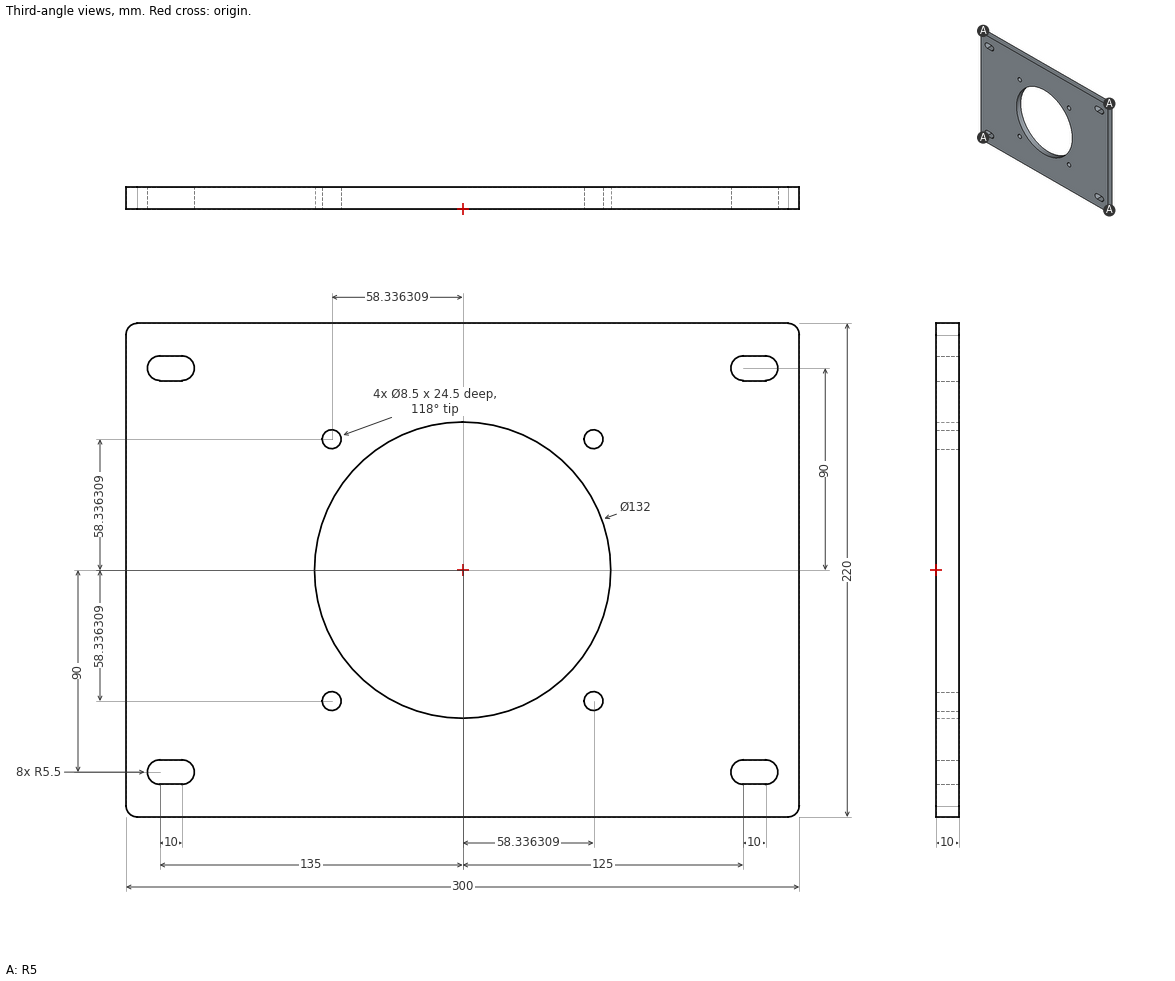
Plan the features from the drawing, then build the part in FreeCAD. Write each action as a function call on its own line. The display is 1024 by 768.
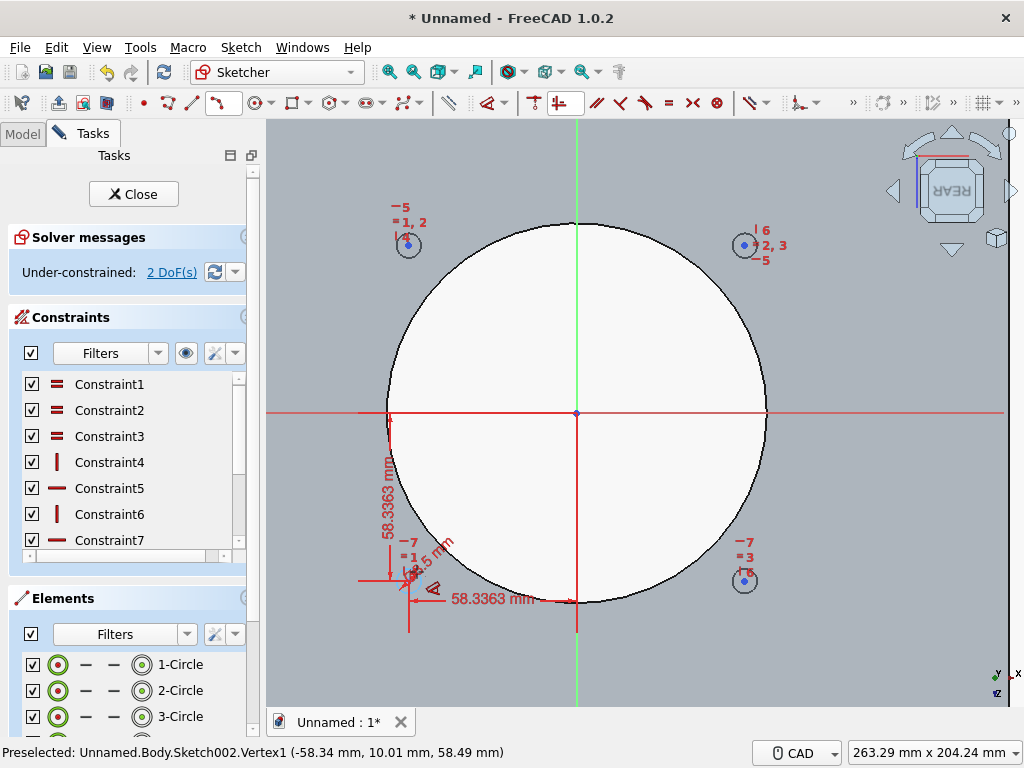
click(409, 246)
click(375, 329)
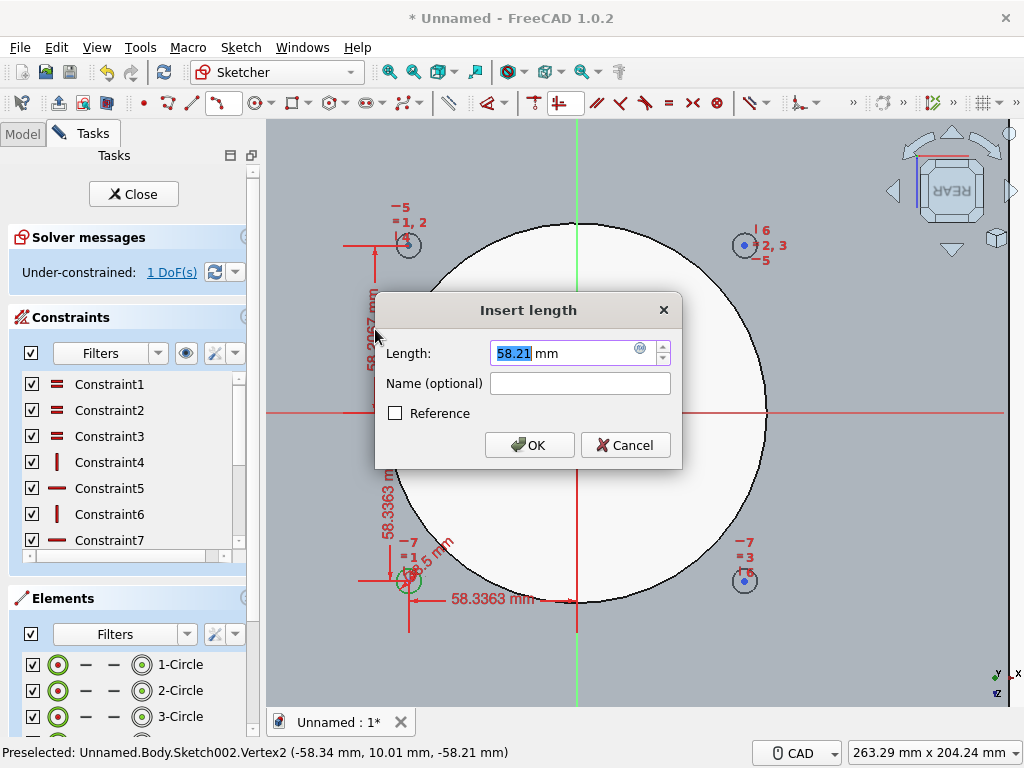
text(58.336309)
key(Return)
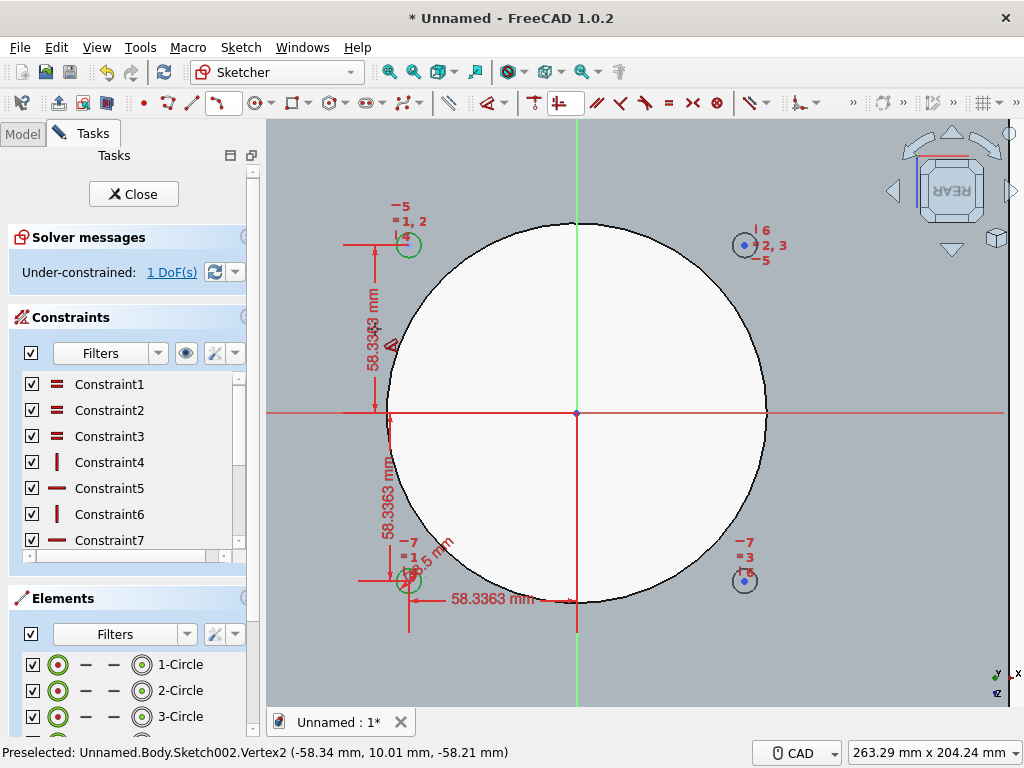
click(745, 245)
click(661, 211)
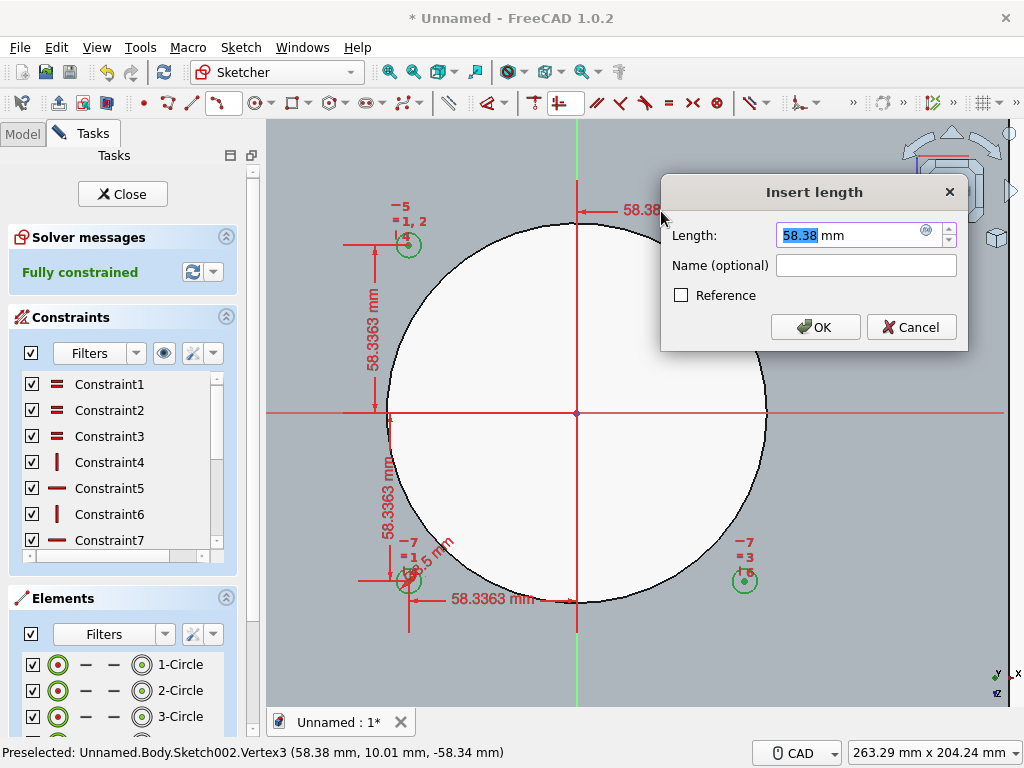
text(58.336309)
key(Return)
key(Escape)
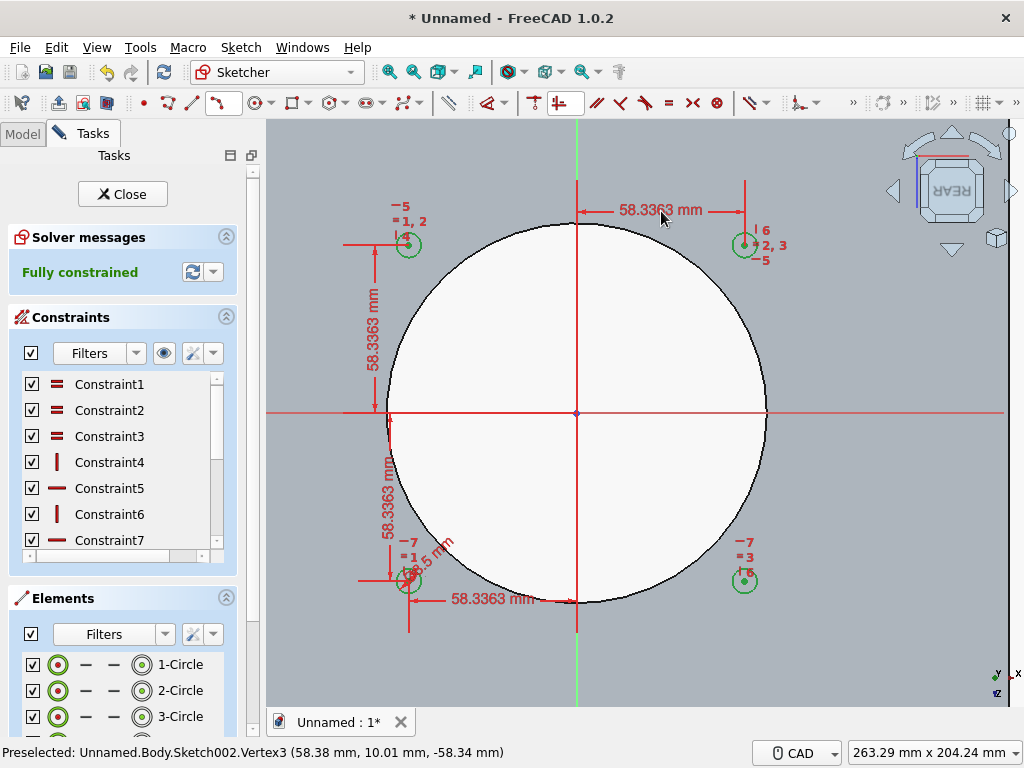
click(123, 194)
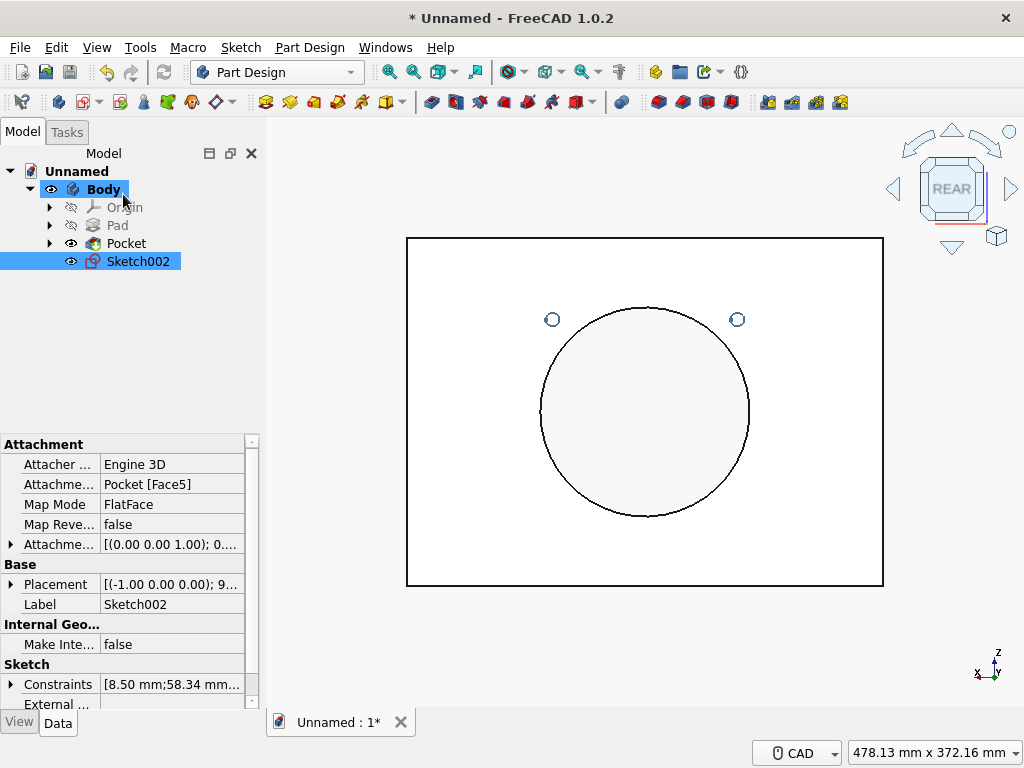
click(456, 102)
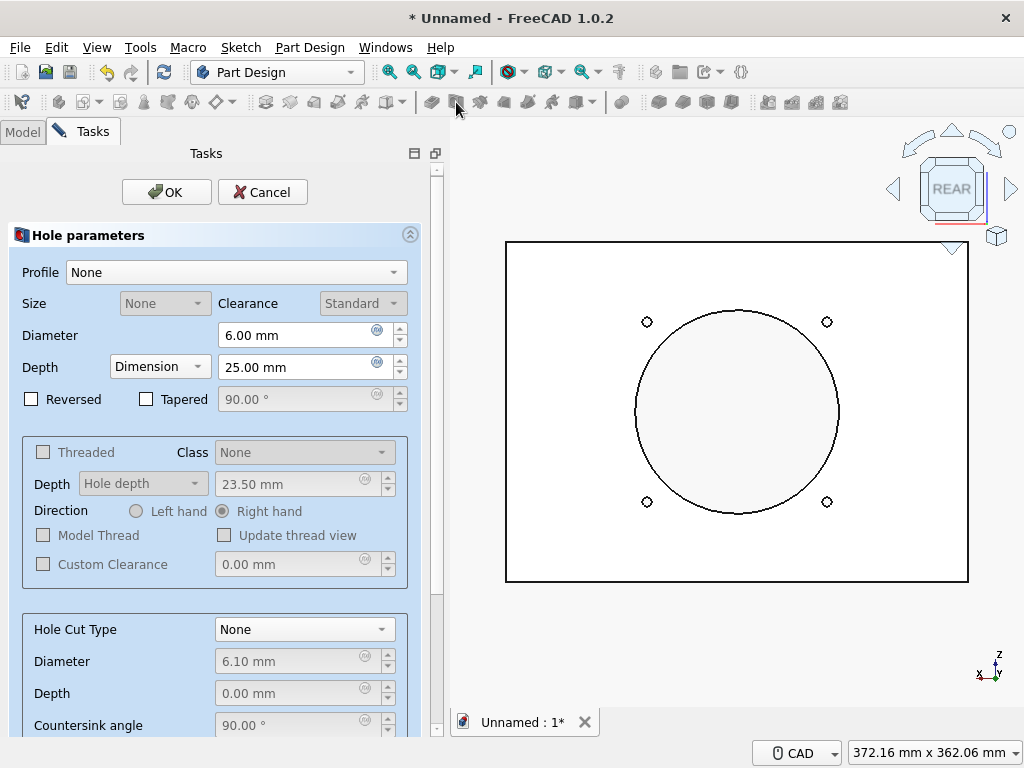
triple_click(305, 335)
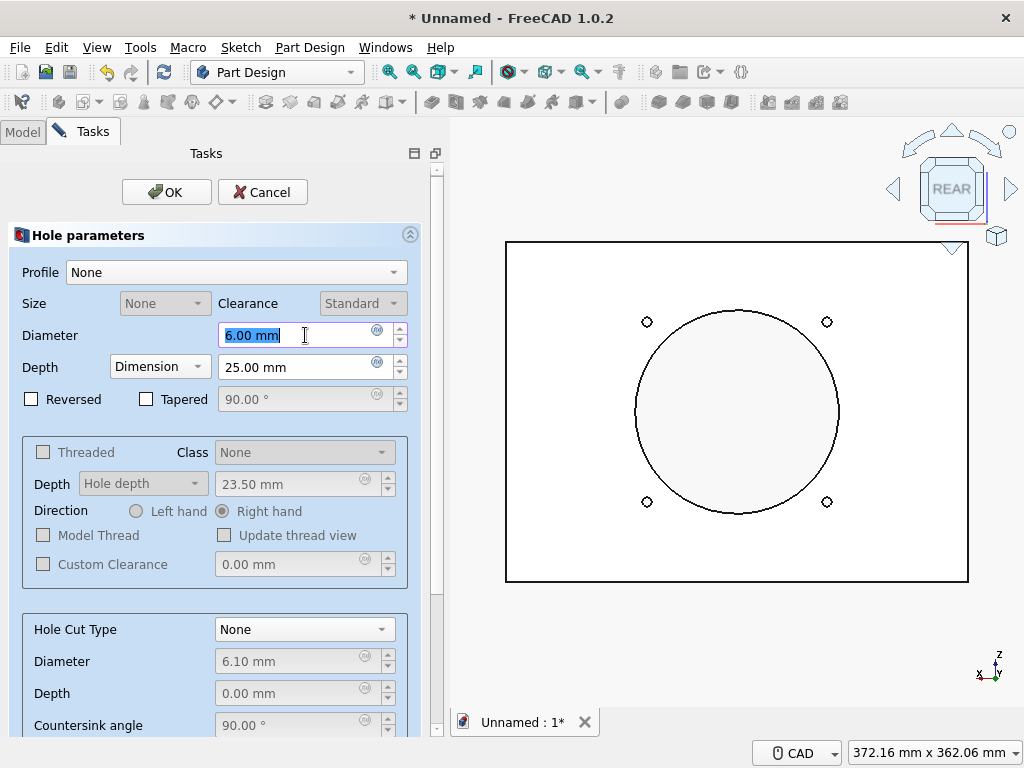
text(8.5)
key(Tab)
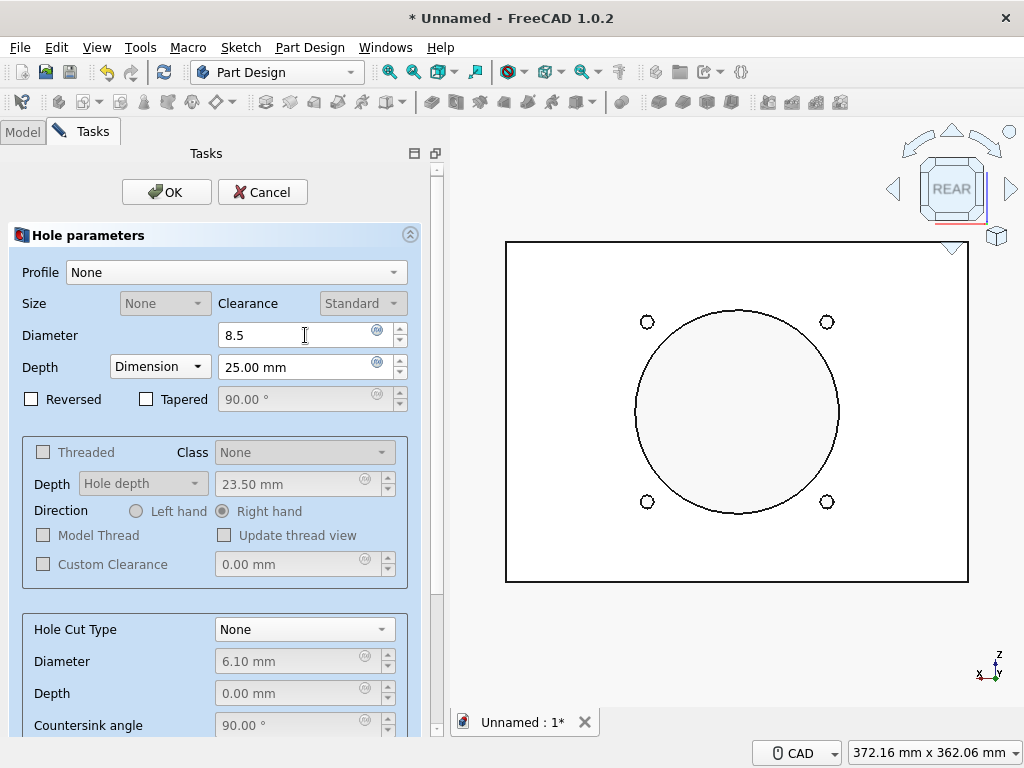
triple_click(305, 367)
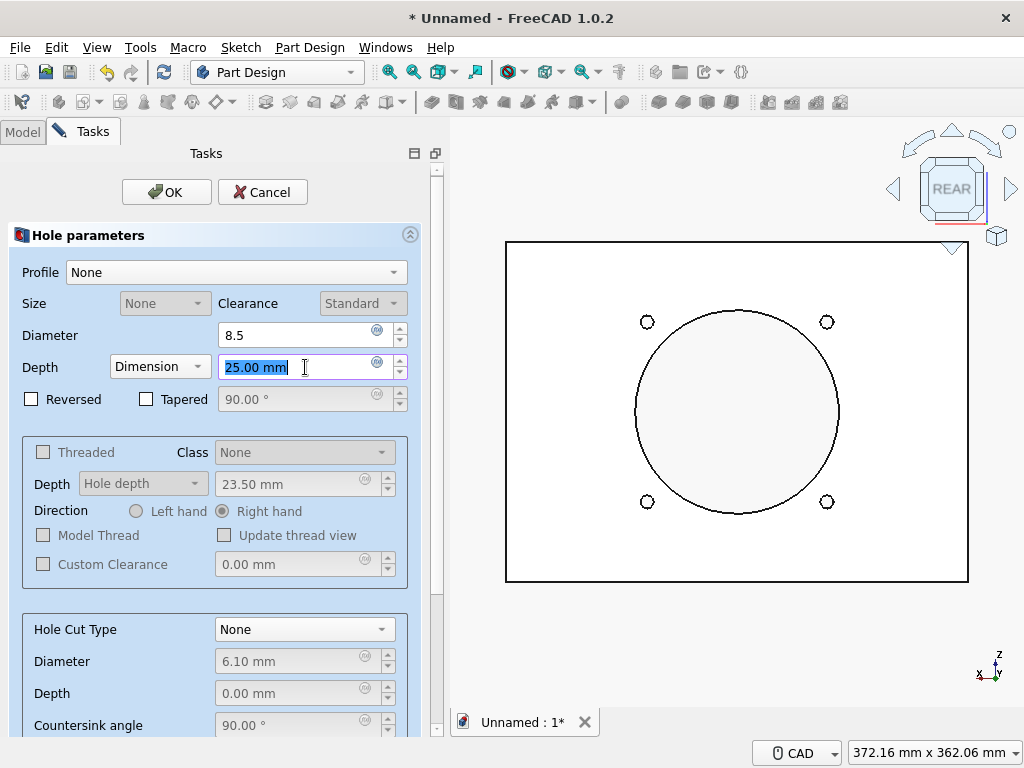
text(24.5)
key(Tab)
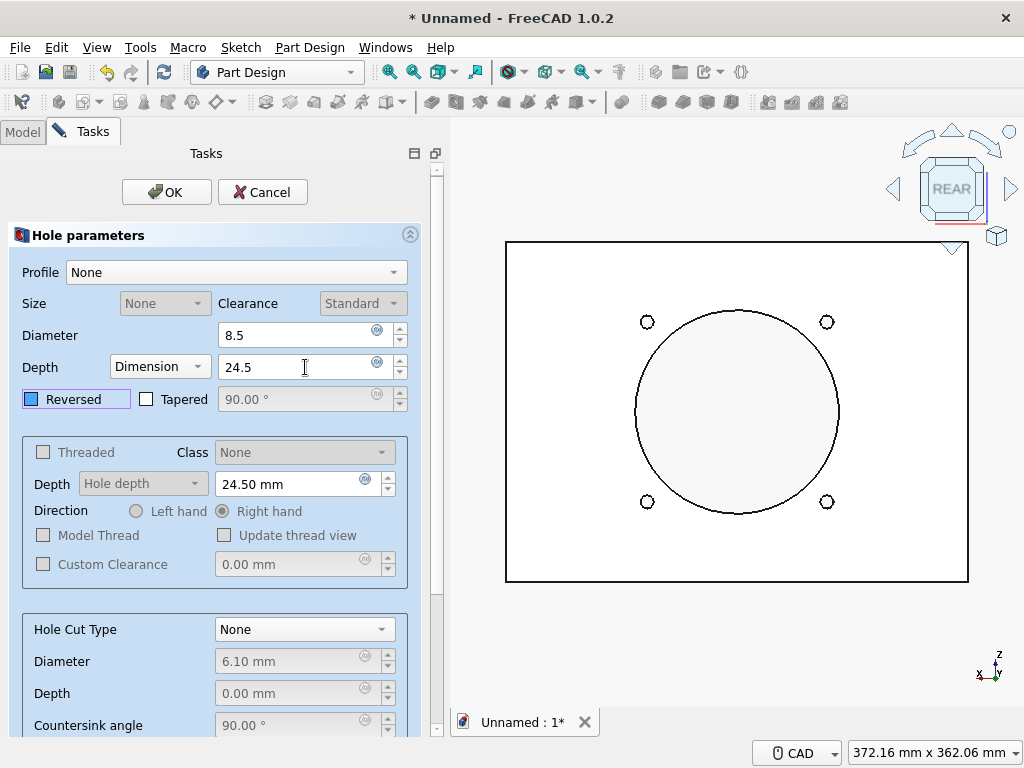
click(167, 192)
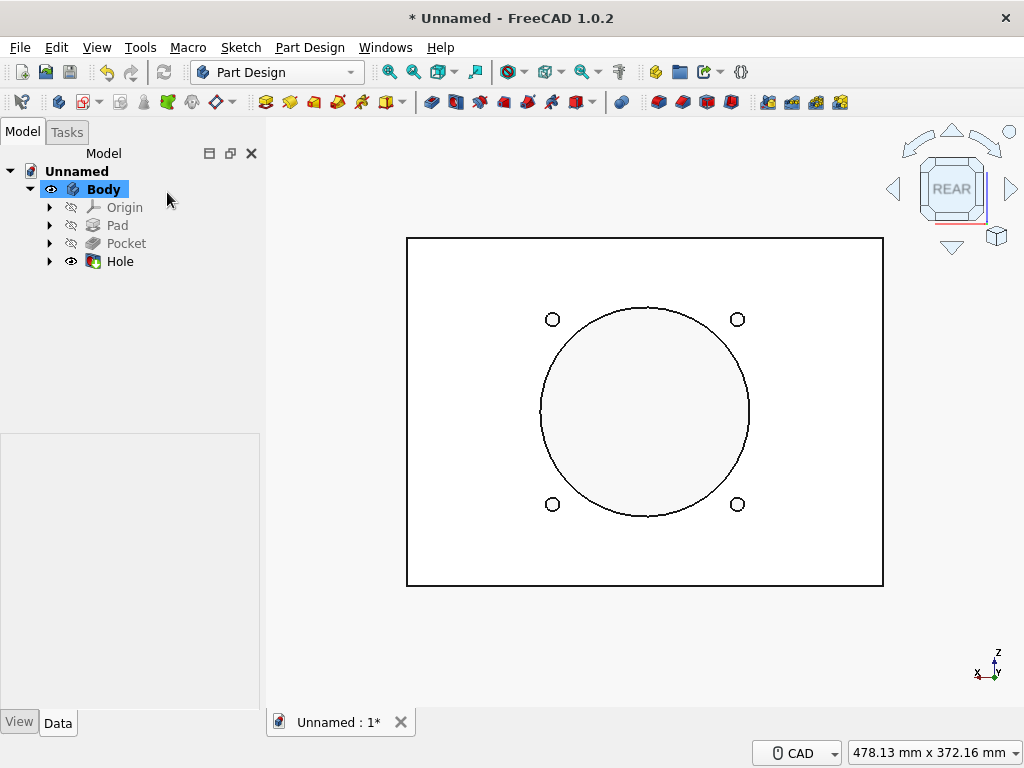
click(509, 461)